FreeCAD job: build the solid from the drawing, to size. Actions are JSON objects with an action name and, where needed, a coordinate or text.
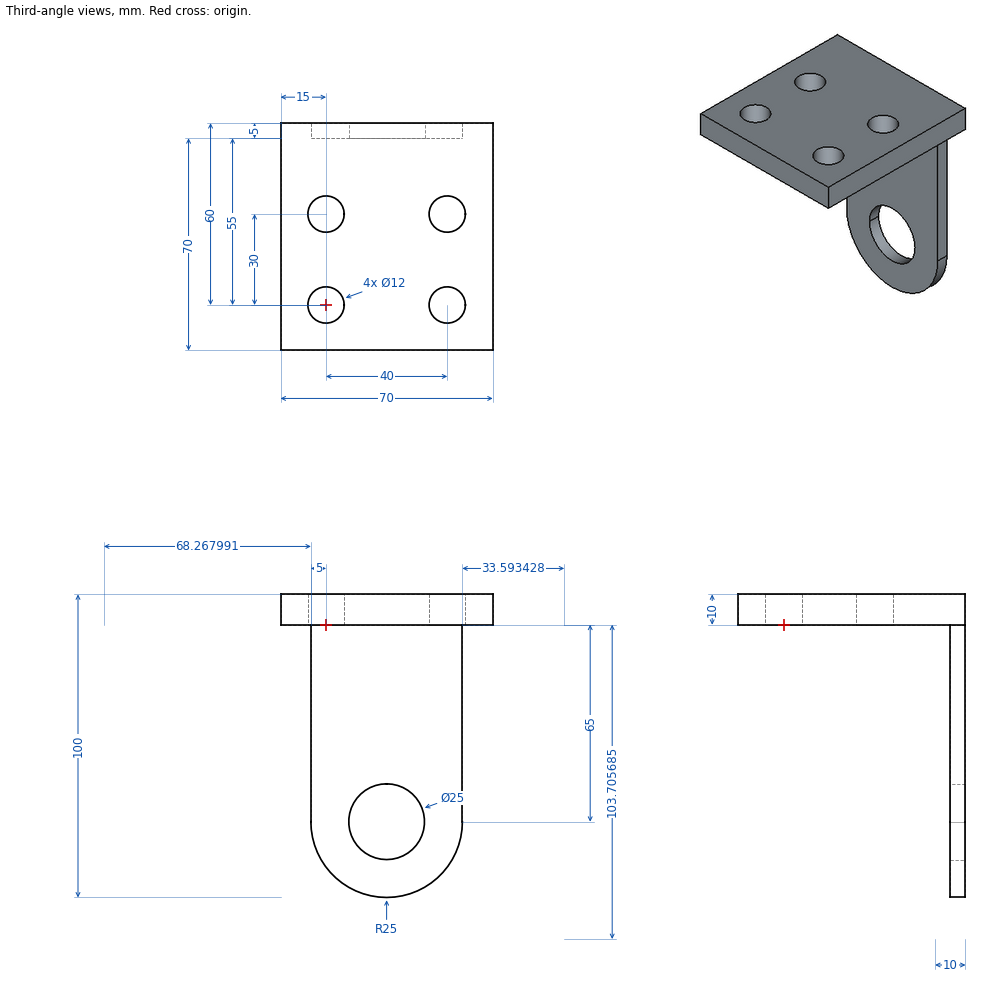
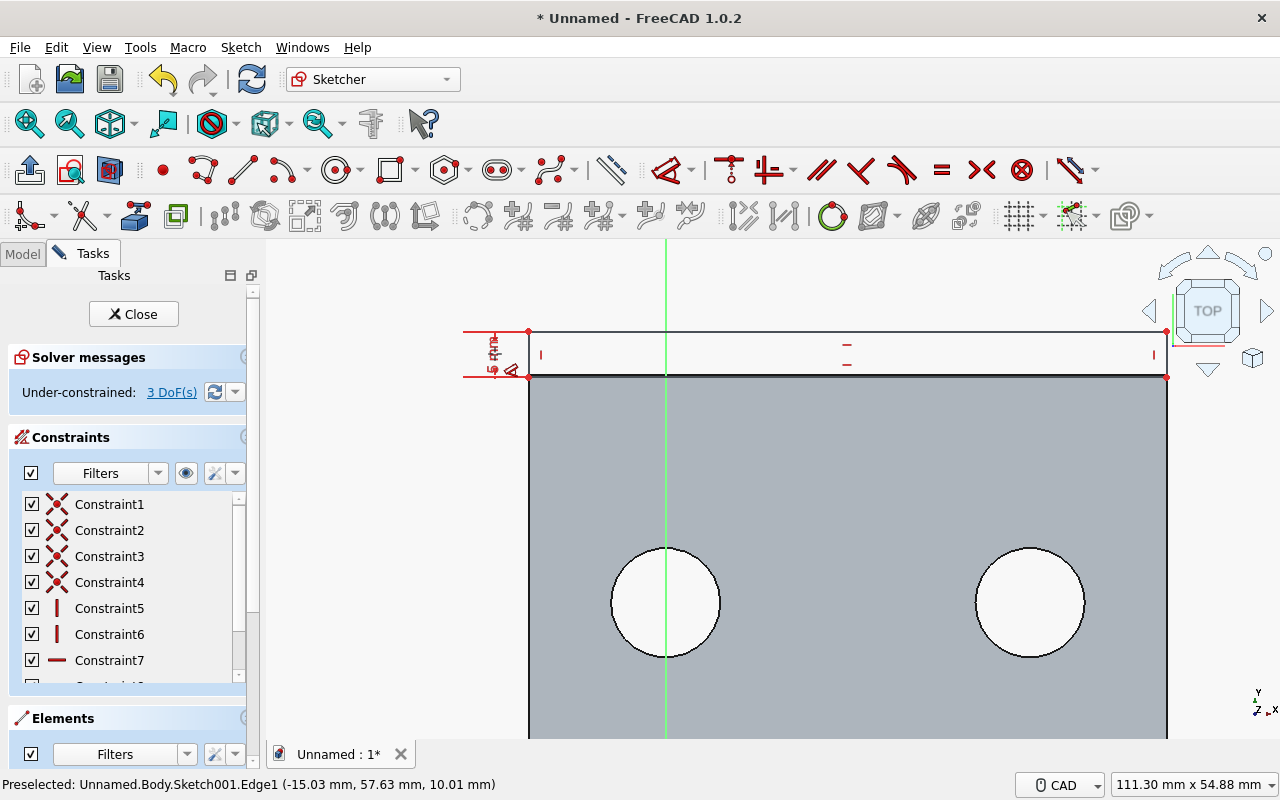
{"action": "left_click", "coordinate": [720, 377]}
{"action": "left_click", "coordinate": [822, 411]}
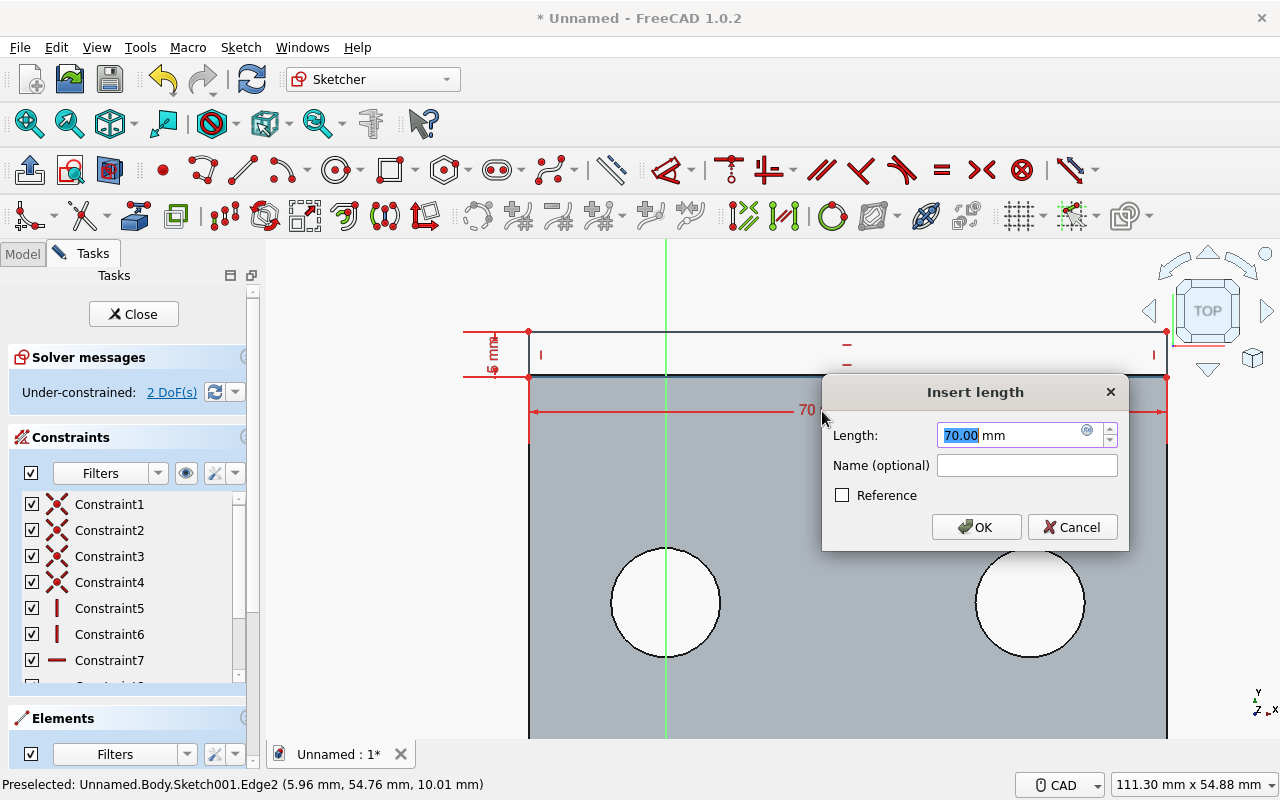
{"action": "type", "text": "70"}
{"action": "key", "text": "Return"}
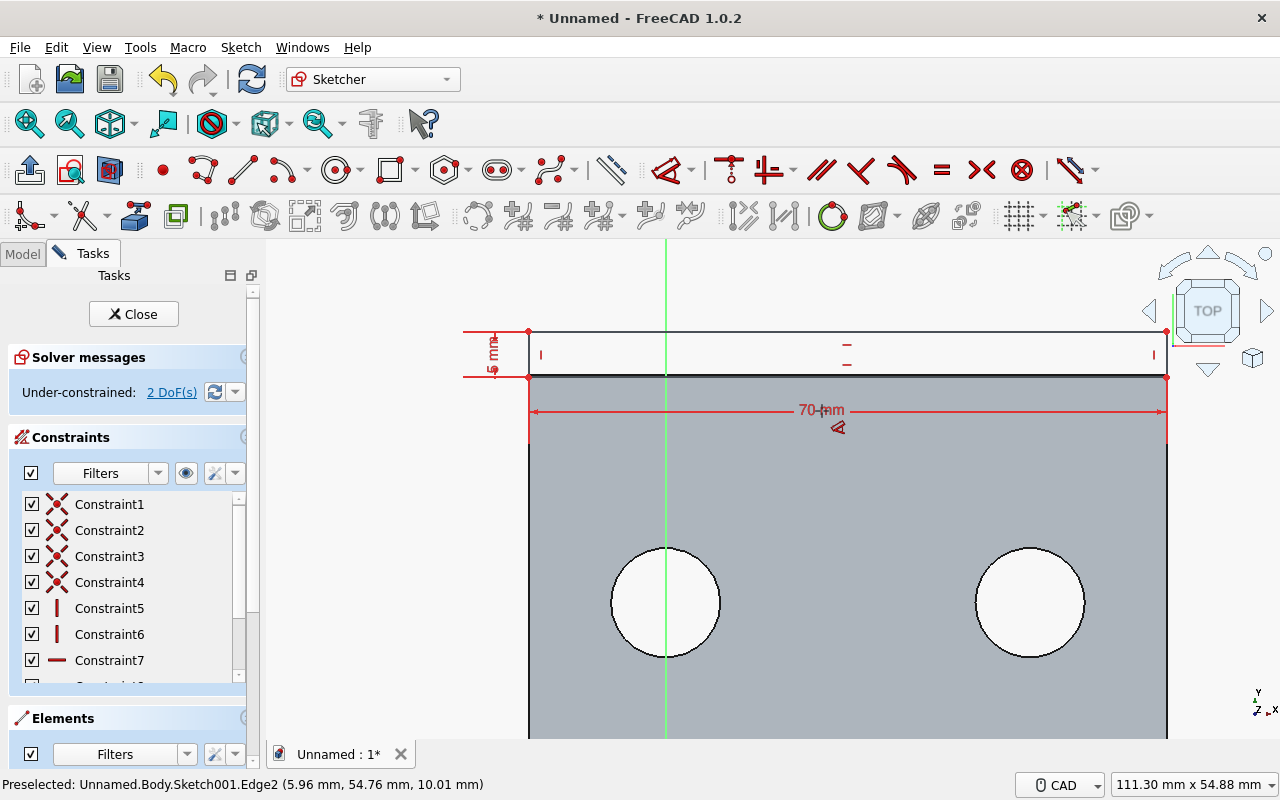
{"action": "left_click", "coordinate": [529, 332]}
{"action": "left_click", "coordinate": [597, 298]}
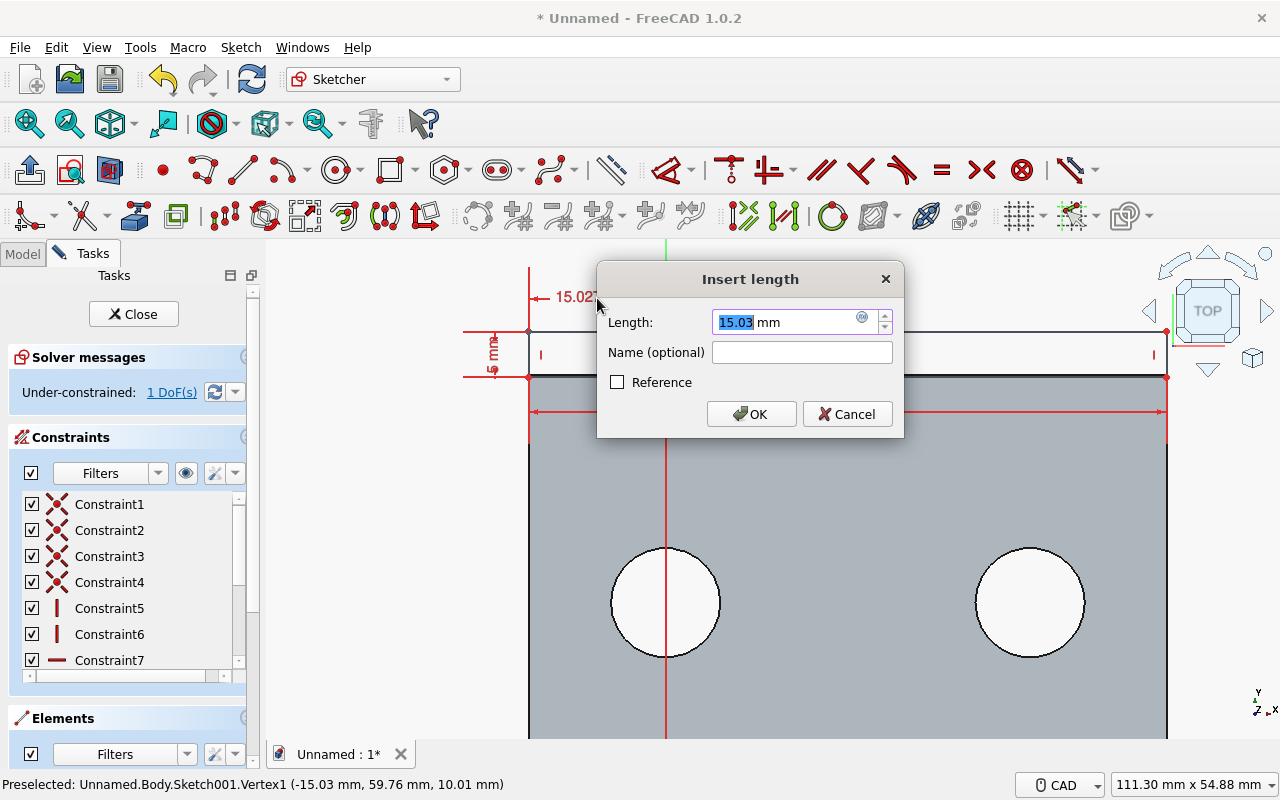
{"action": "type", "text": "15"}
{"action": "key", "text": "Return"}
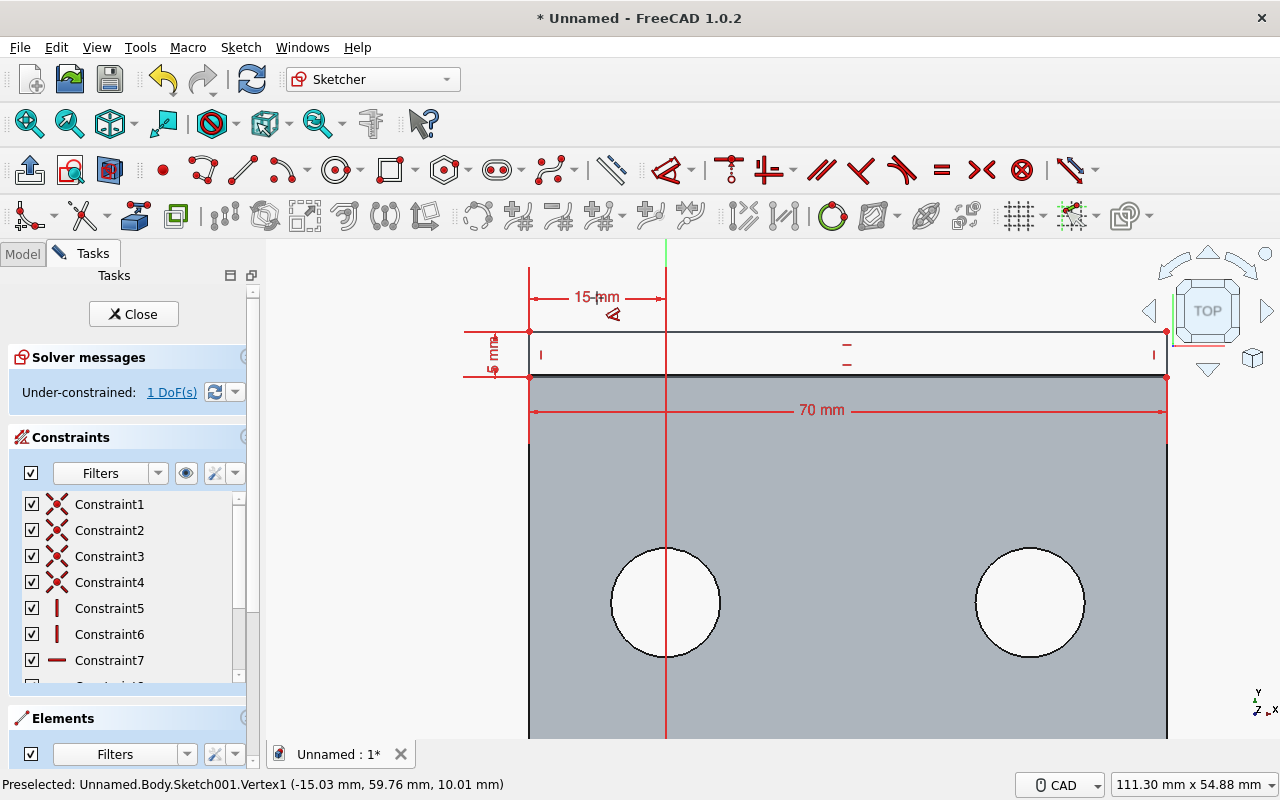
{"action": "left_click", "coordinate": [529, 332]}
{"action": "left_click", "coordinate": [495, 521]}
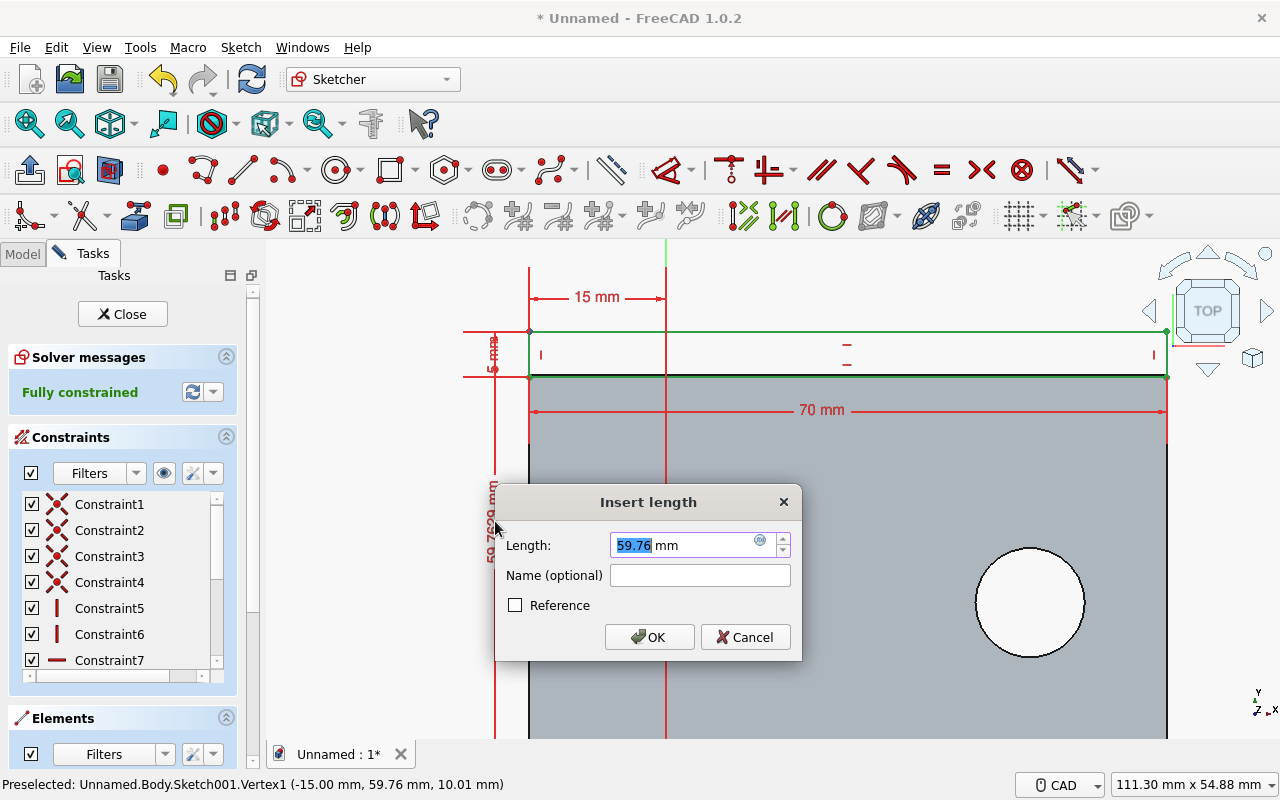
{"action": "type", "text": "60"}
{"action": "key", "text": "Return"}
{"action": "key", "text": "Escape"}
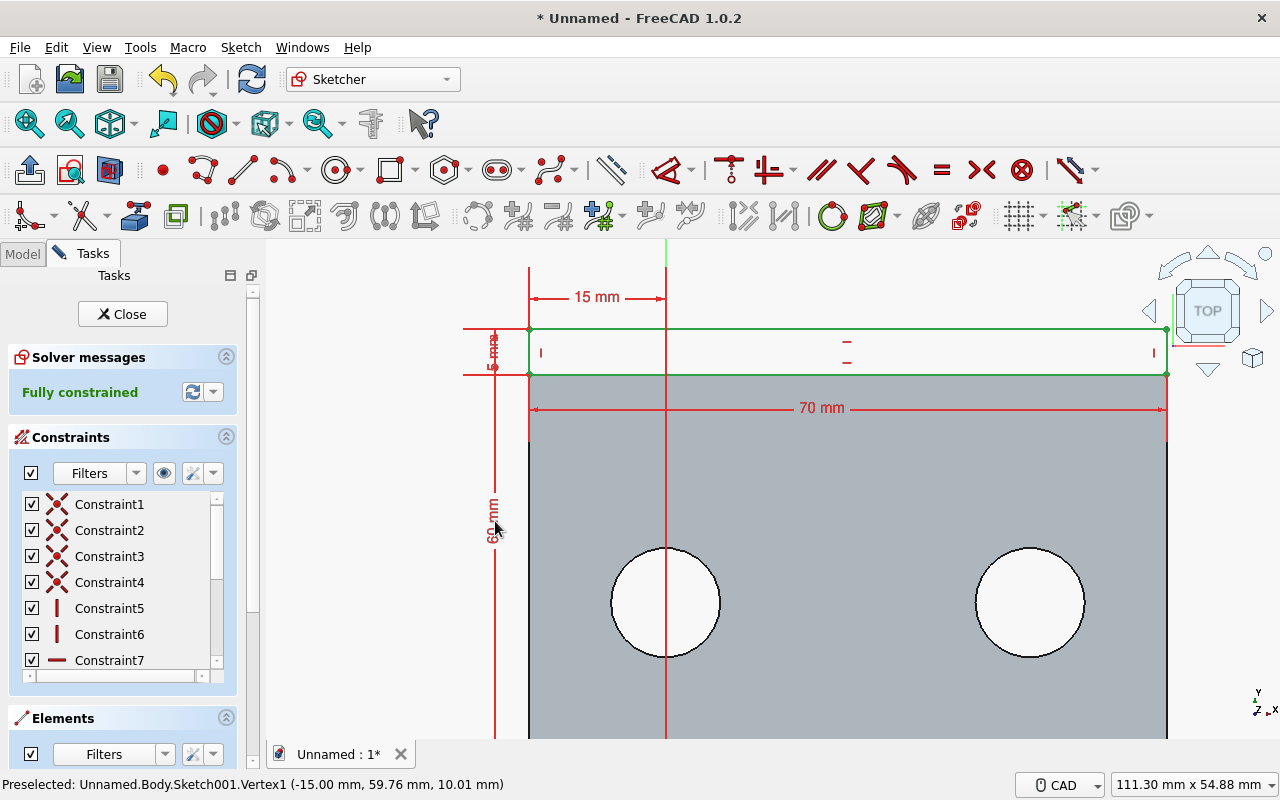
{"action": "left_click", "coordinate": [123, 314]}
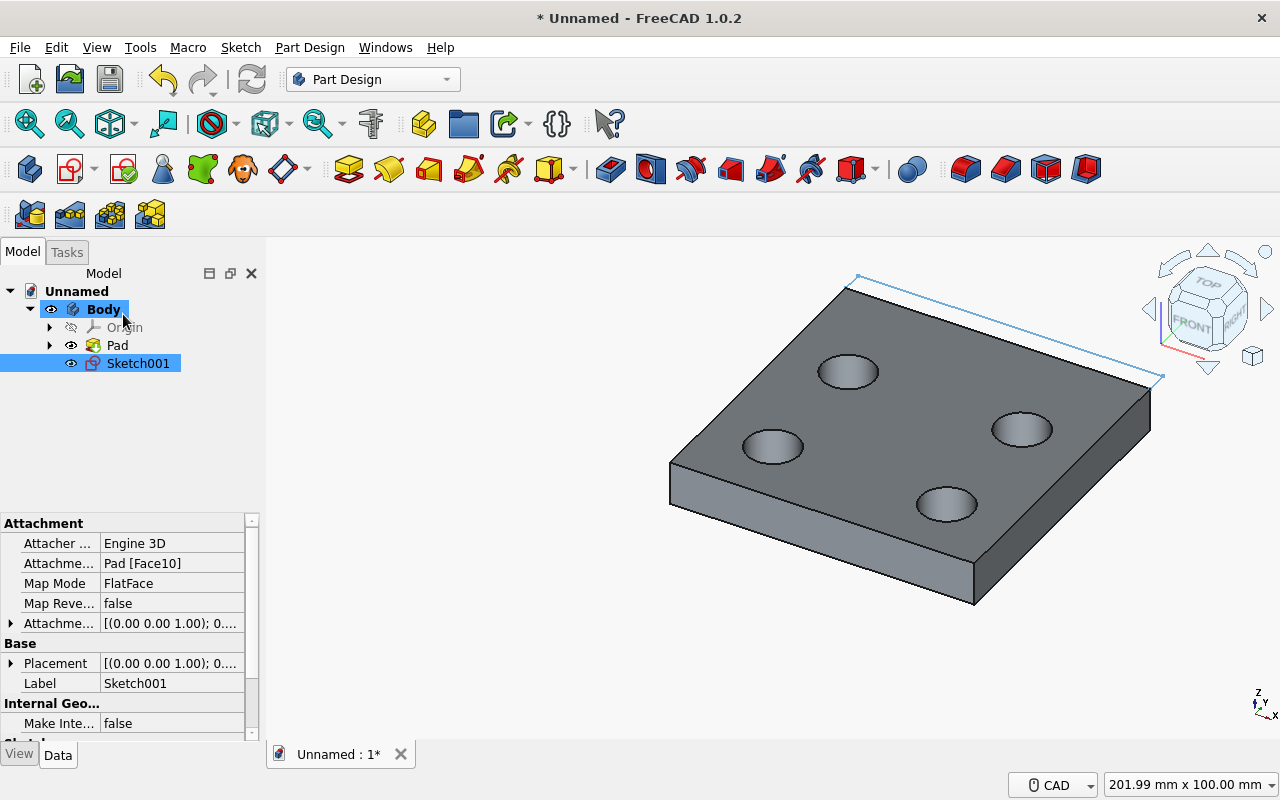
{"action": "left_click", "coordinate": [350, 170]}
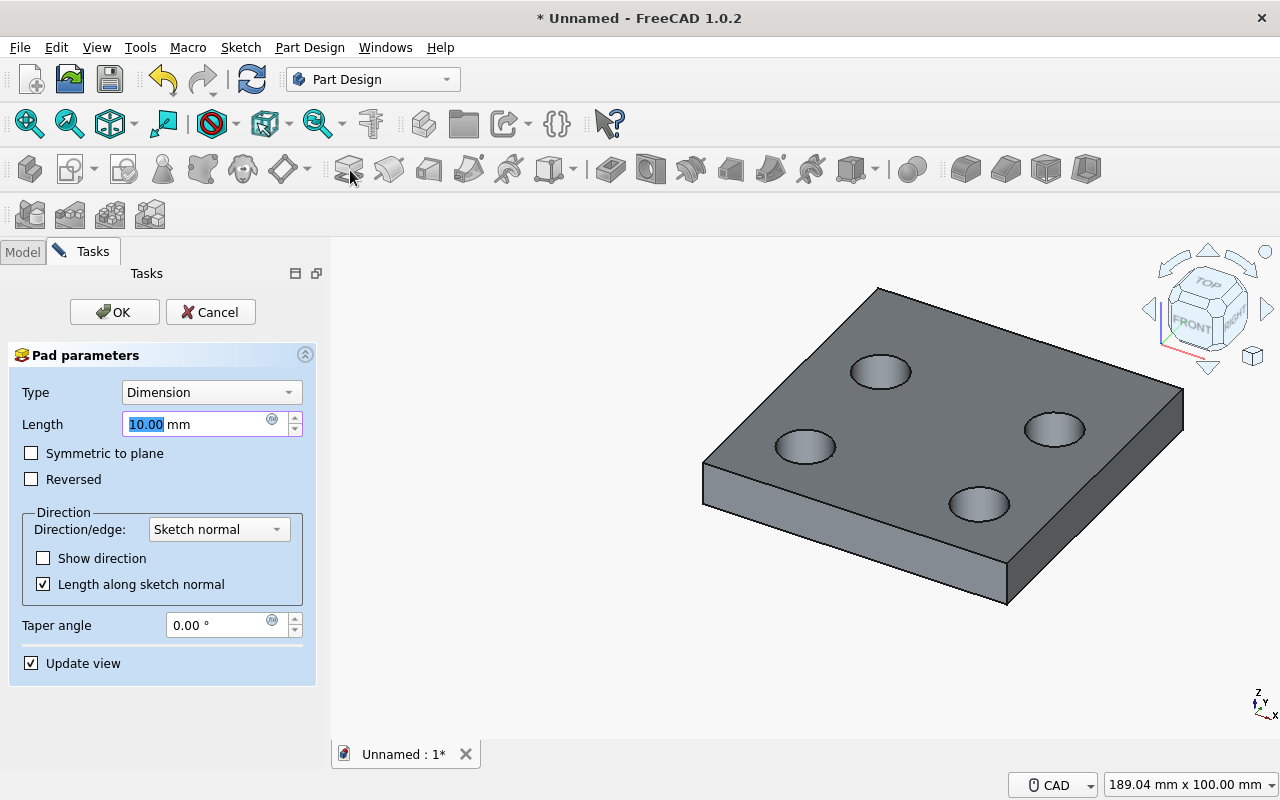
{"action": "type", "text": "100"}
{"action": "key", "text": "Tab"}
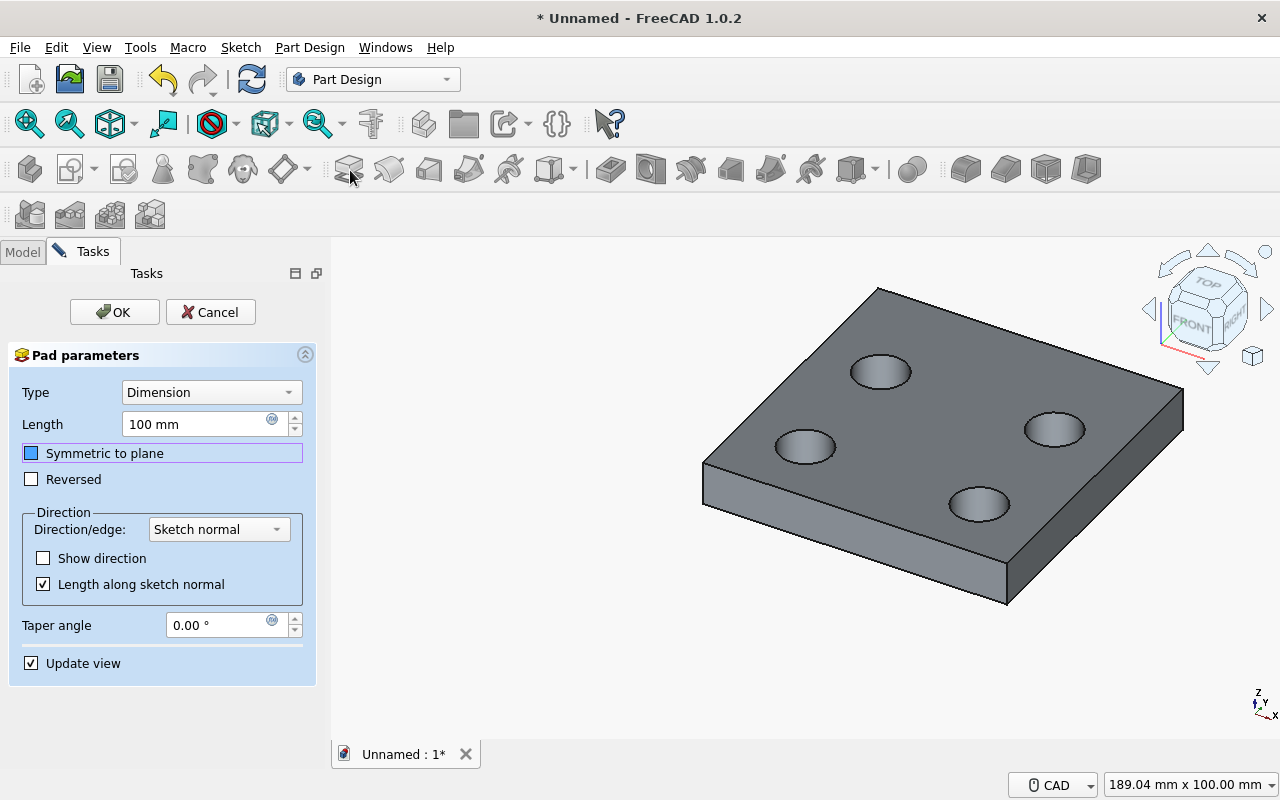
{"action": "left_click", "coordinate": [30, 479]}